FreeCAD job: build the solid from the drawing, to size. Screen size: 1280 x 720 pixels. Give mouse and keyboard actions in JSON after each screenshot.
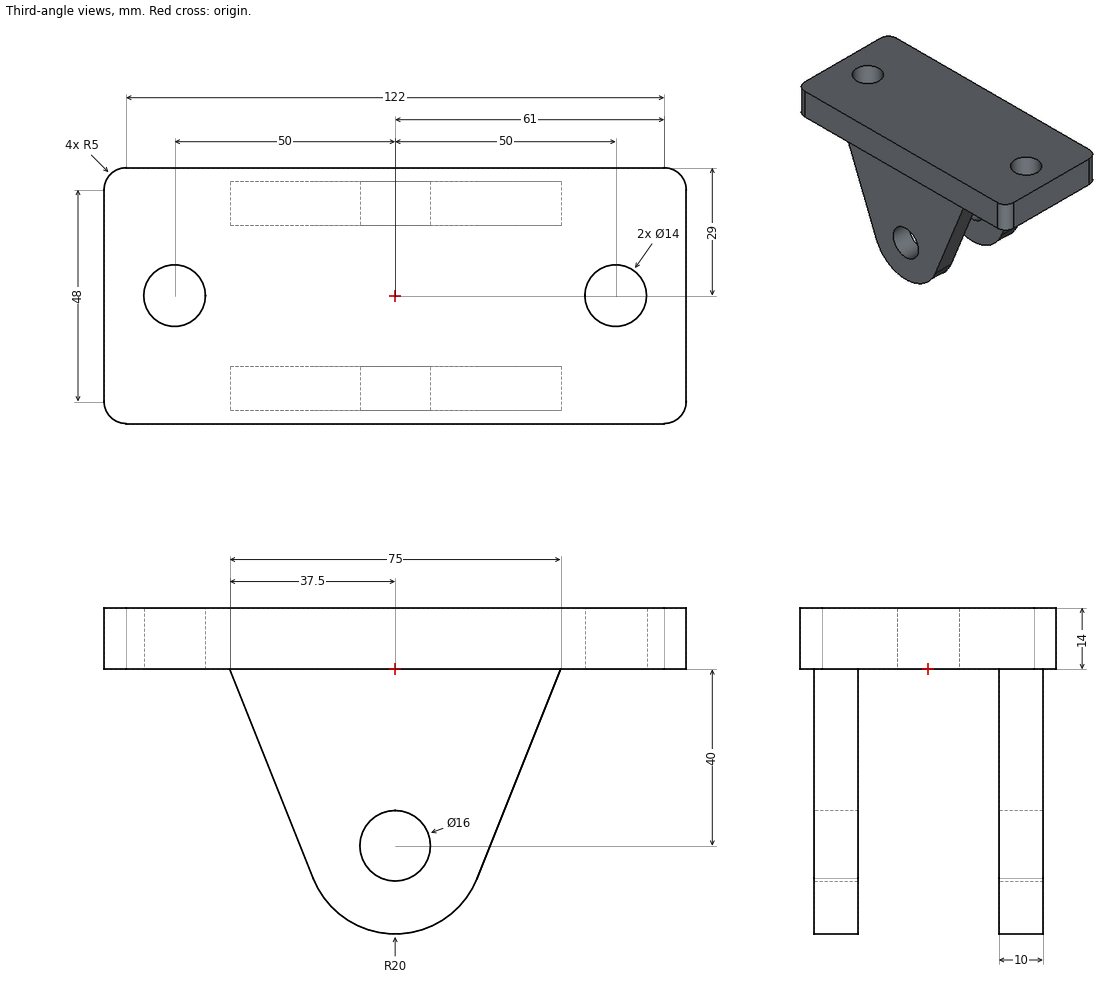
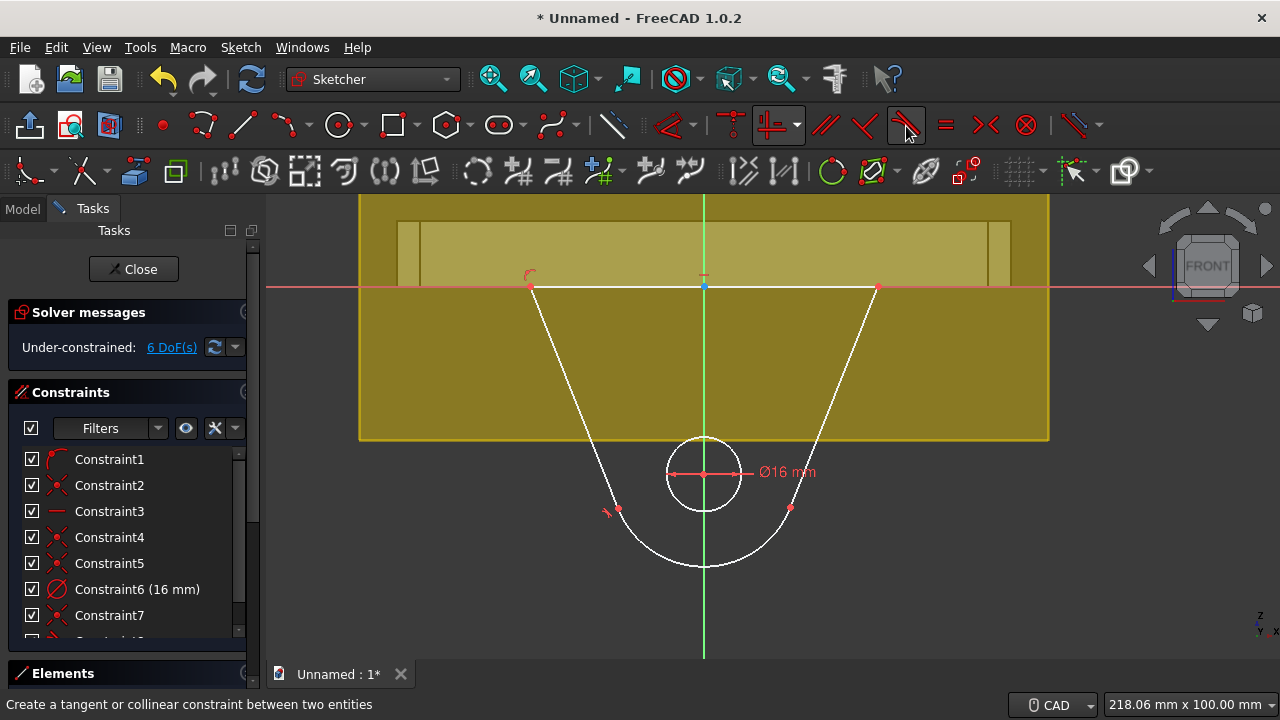
{"action": "left_click", "coordinate": [852, 353]}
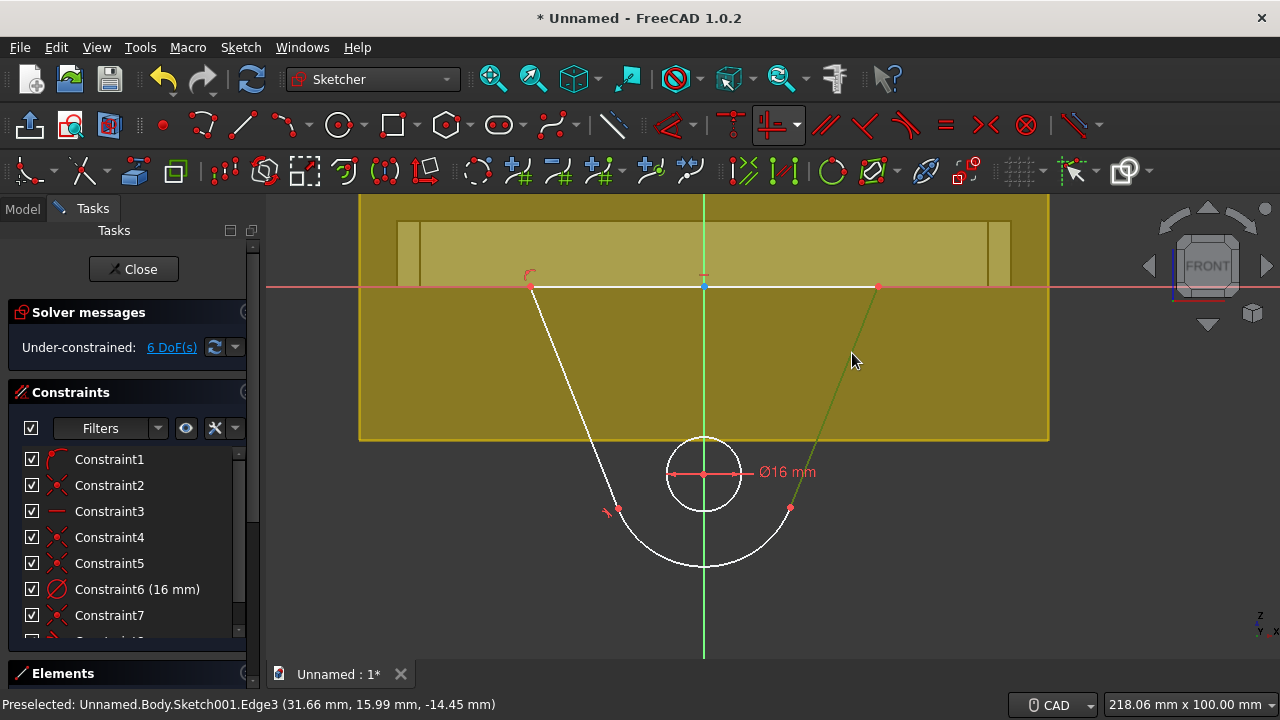
{"action": "left_click", "coordinate": [662, 556]}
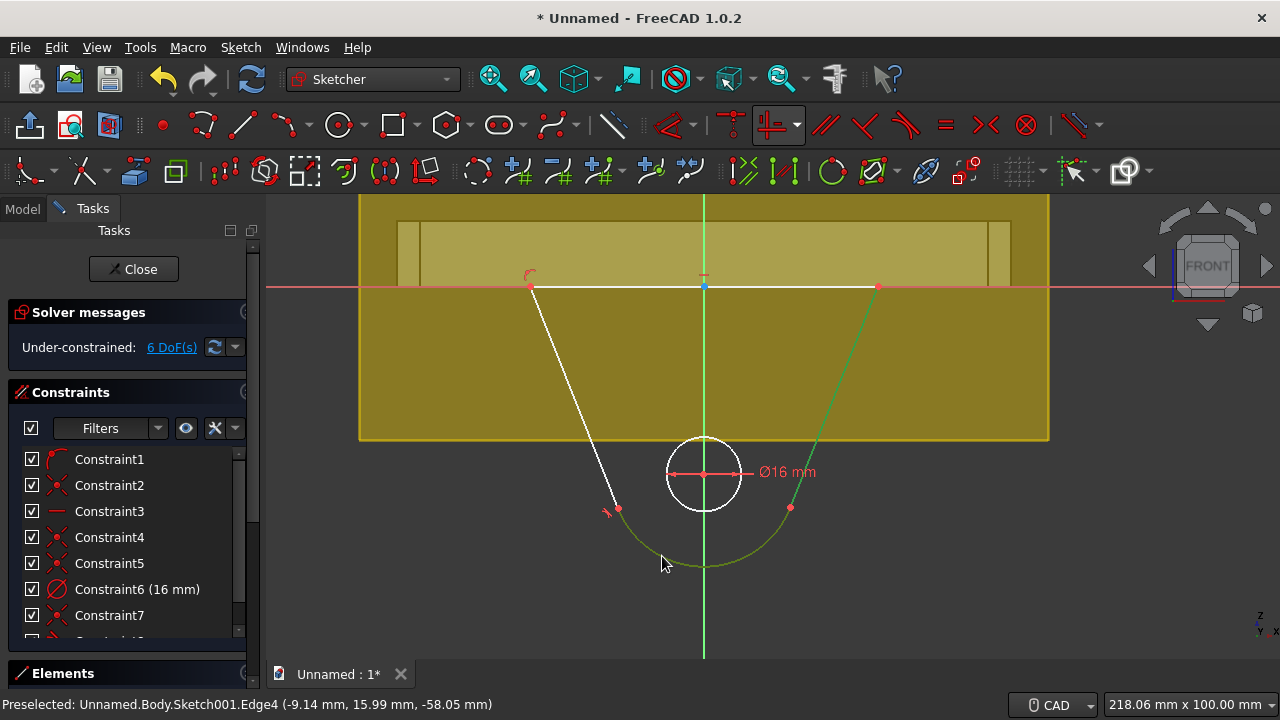
{"action": "left_click", "coordinate": [906, 126]}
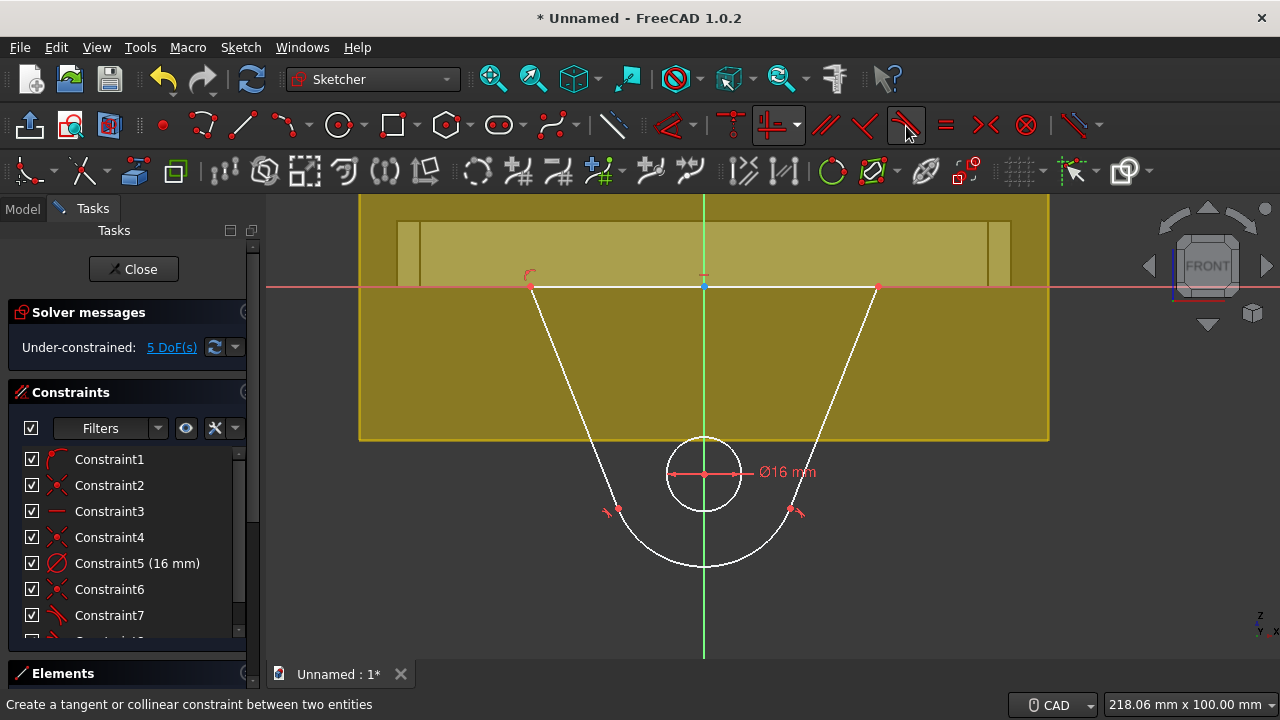
{"action": "left_click", "coordinate": [704, 474]}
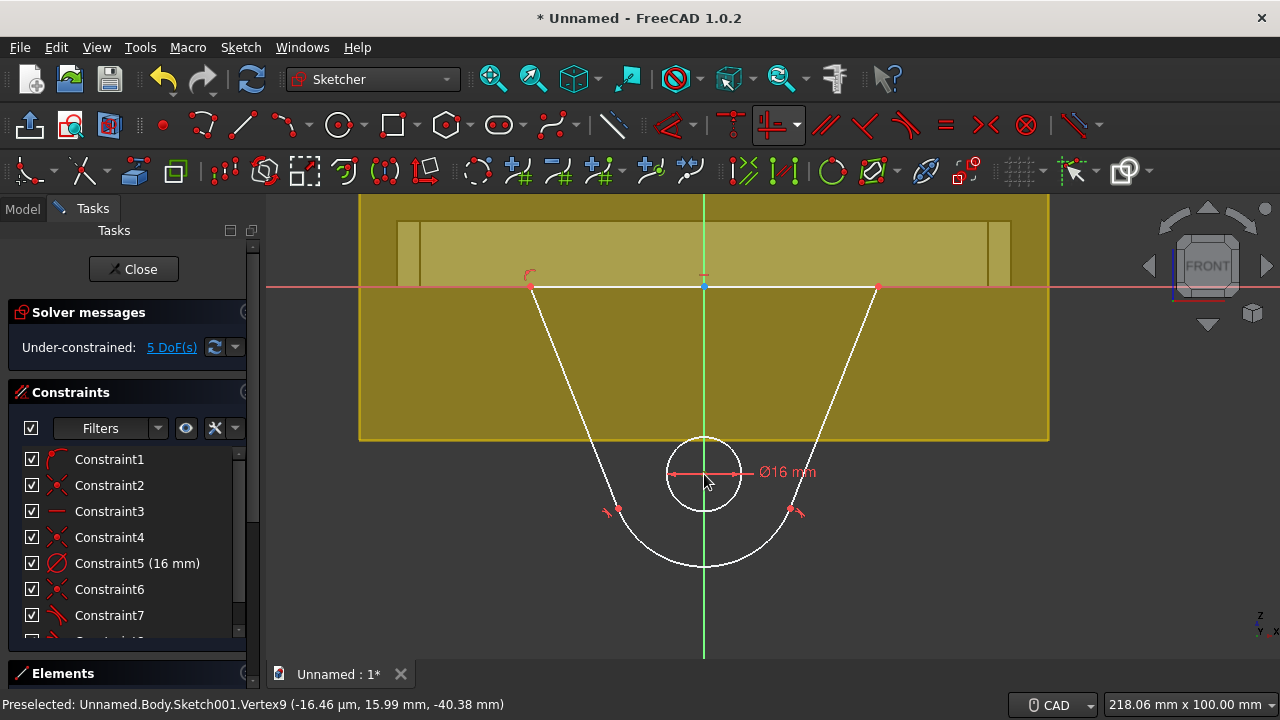
{"action": "left_click", "coordinate": [704, 602]}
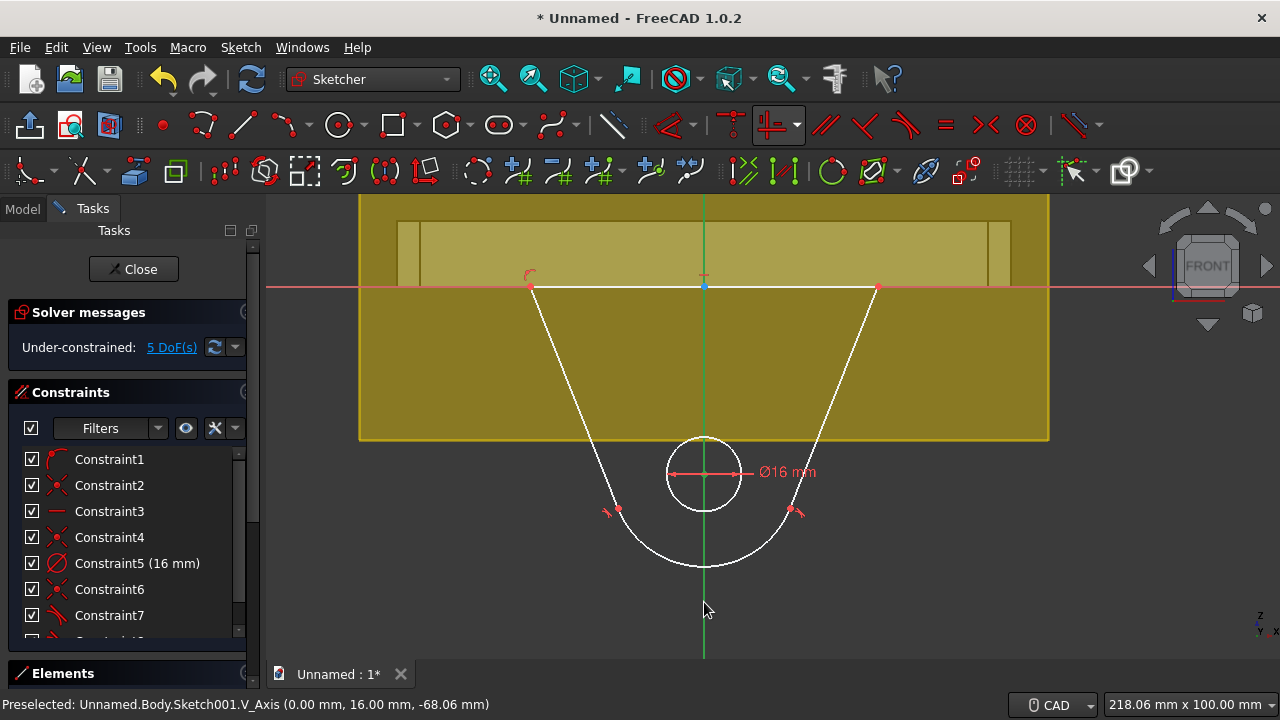
{"action": "left_click", "coordinate": [732, 126]}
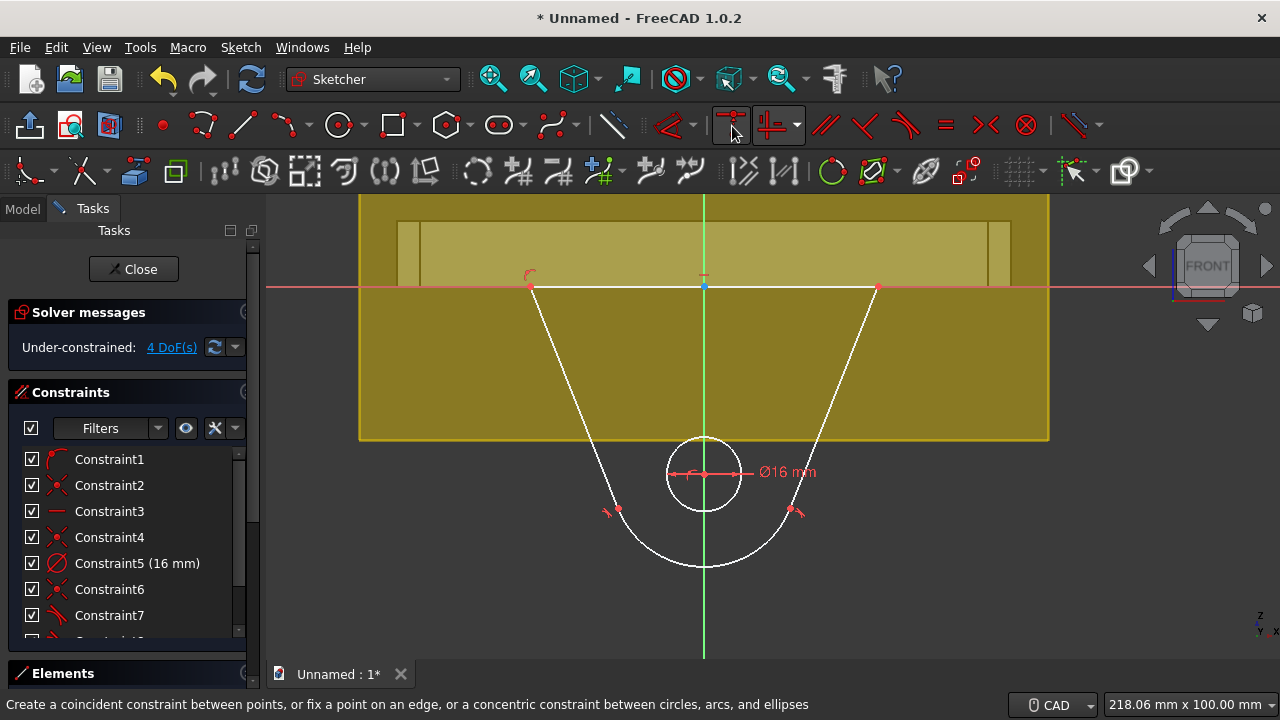
{"action": "left_click", "coordinate": [668, 126]}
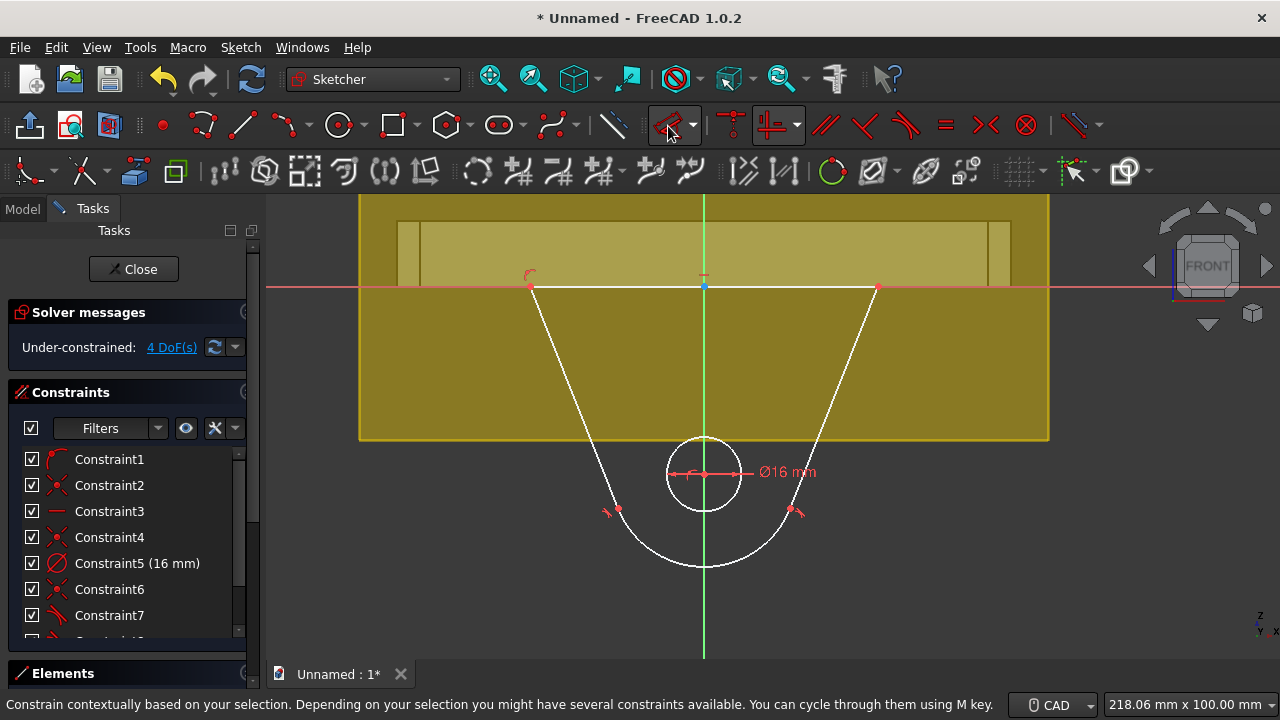
{"action": "left_click", "coordinate": [662, 557]}
{"action": "left_click", "coordinate": [647, 586]}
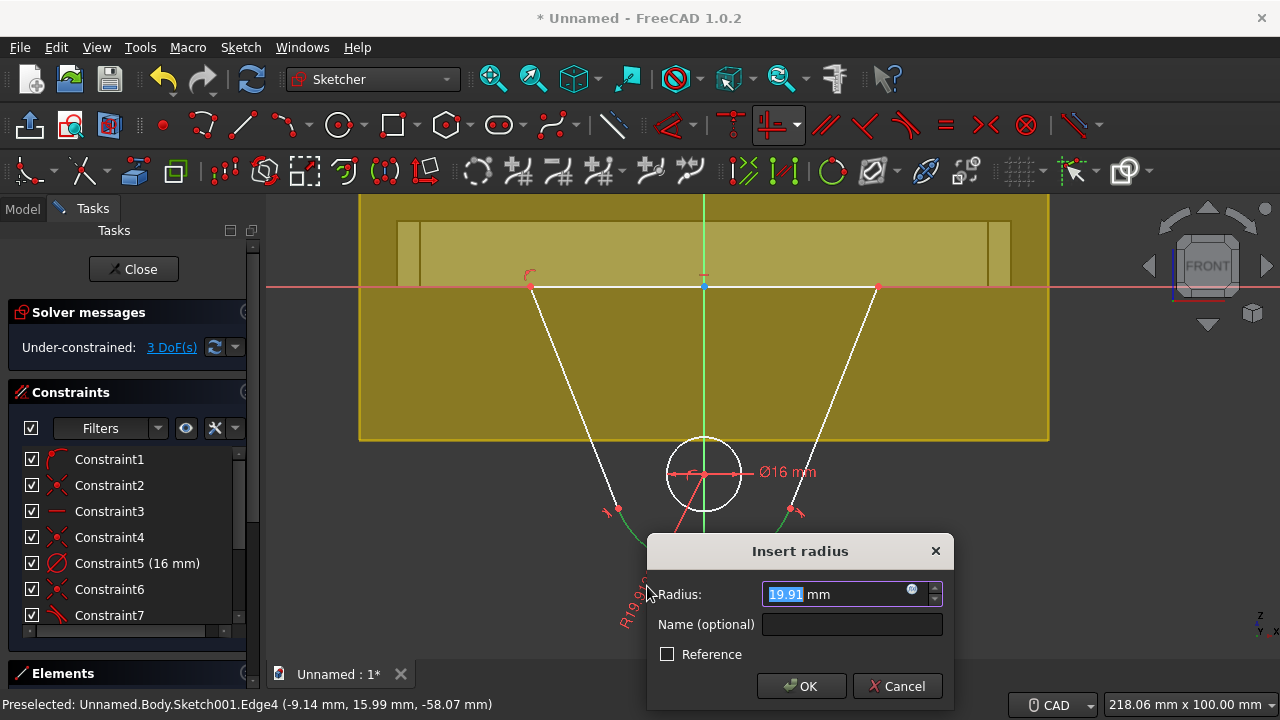
{"action": "type", "text": "20"}
{"action": "key", "text": "Return"}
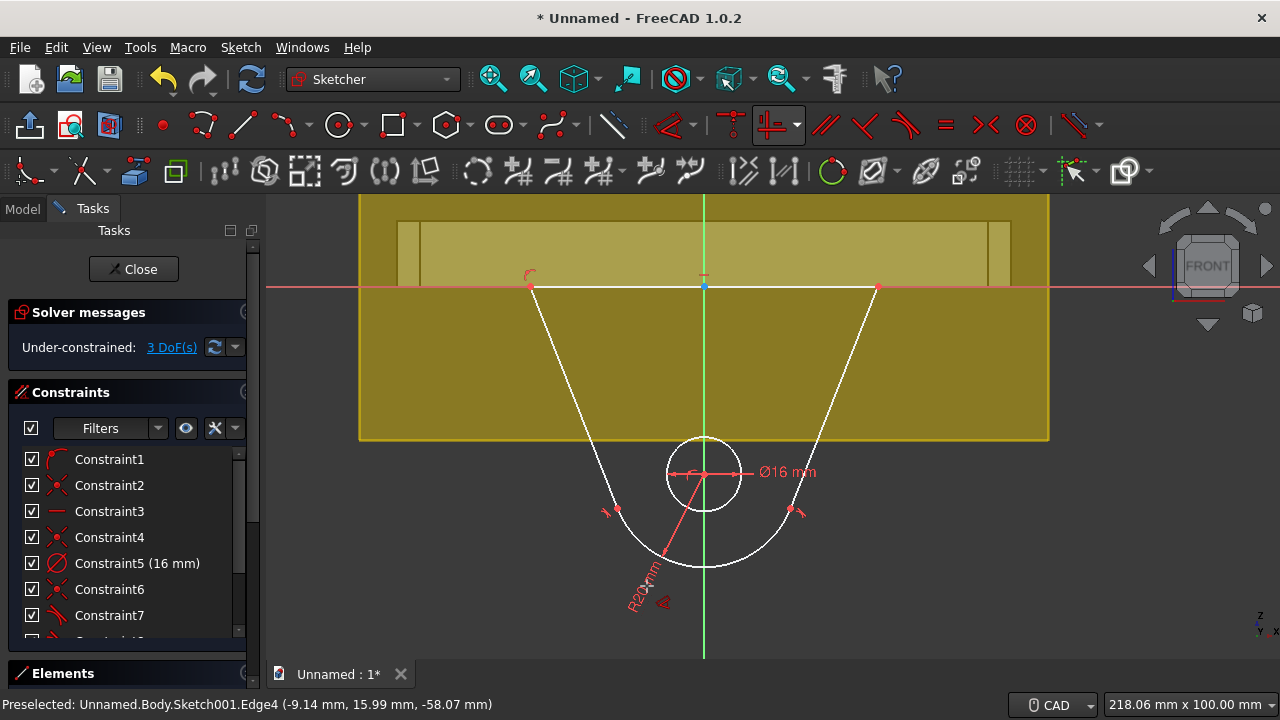
{"action": "left_click", "coordinate": [634, 287]}
{"action": "left_click", "coordinate": [624, 253]}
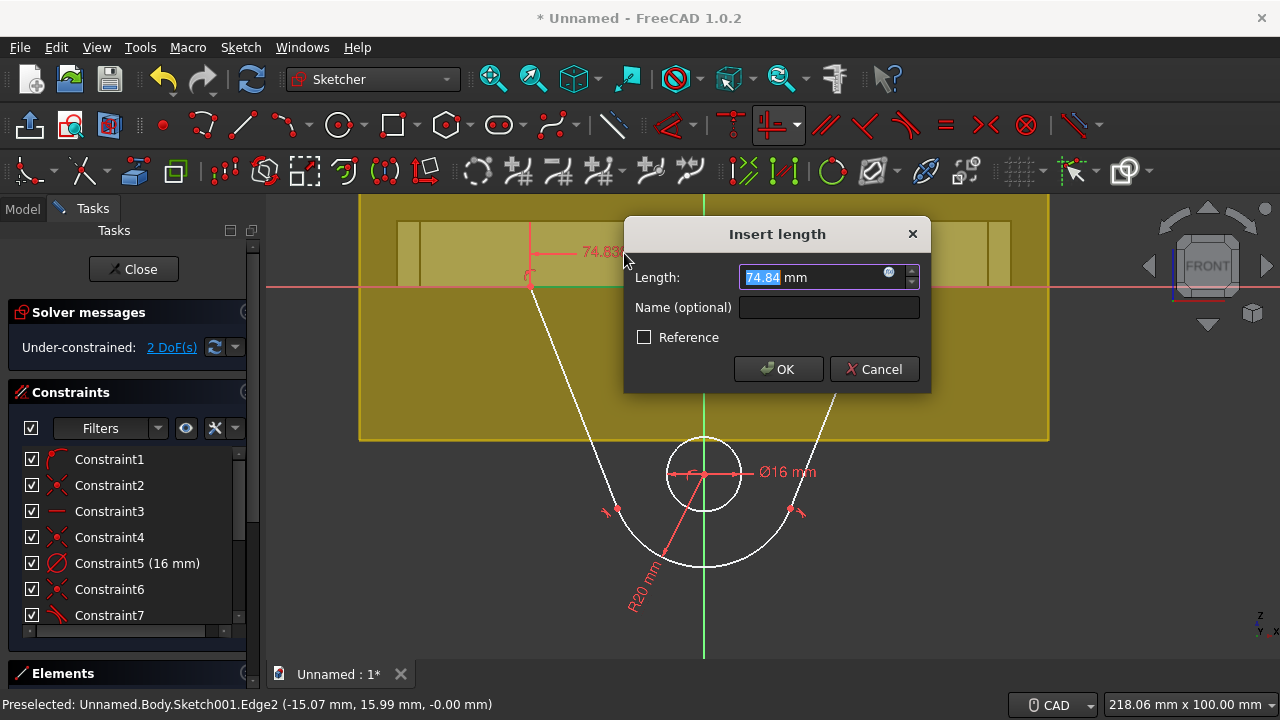
{"action": "type", "text": "75"}
{"action": "key", "text": "Return"}